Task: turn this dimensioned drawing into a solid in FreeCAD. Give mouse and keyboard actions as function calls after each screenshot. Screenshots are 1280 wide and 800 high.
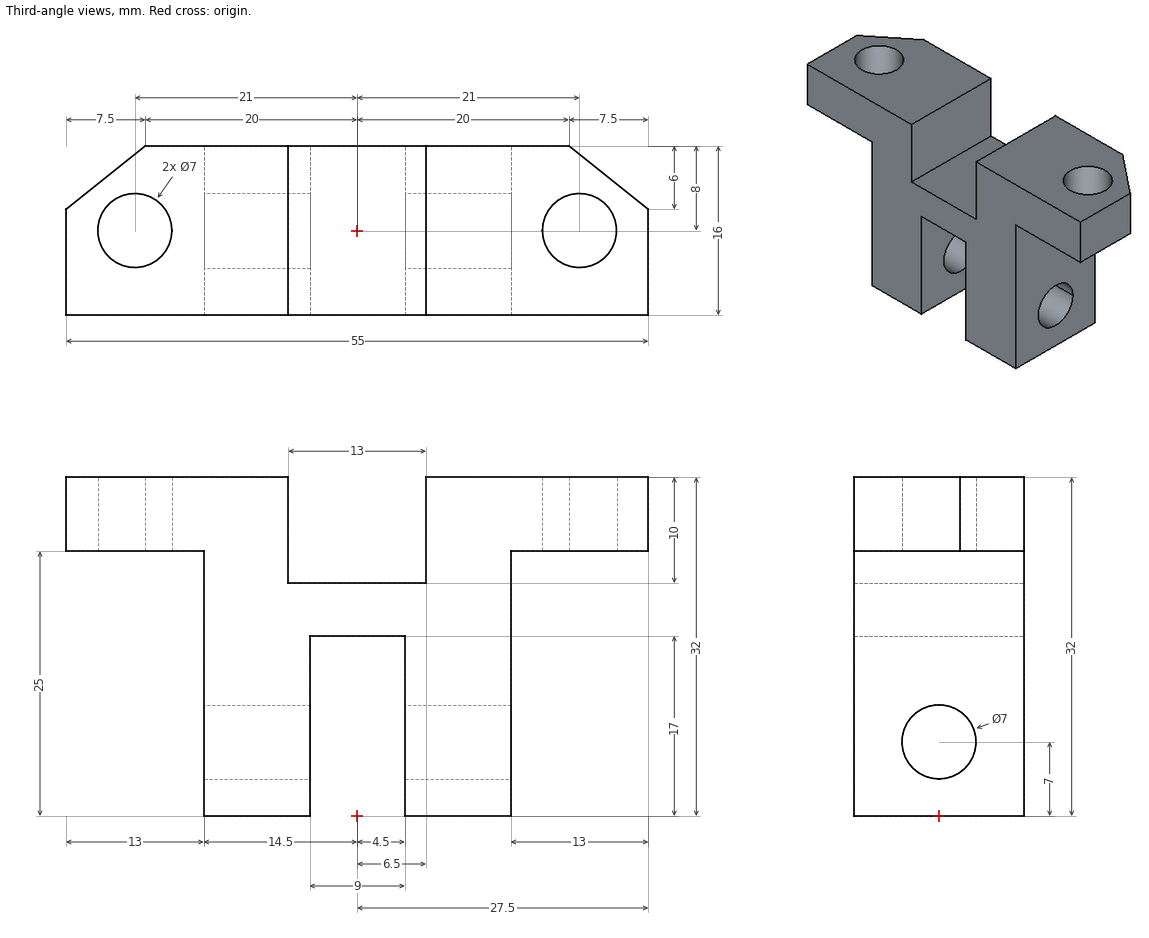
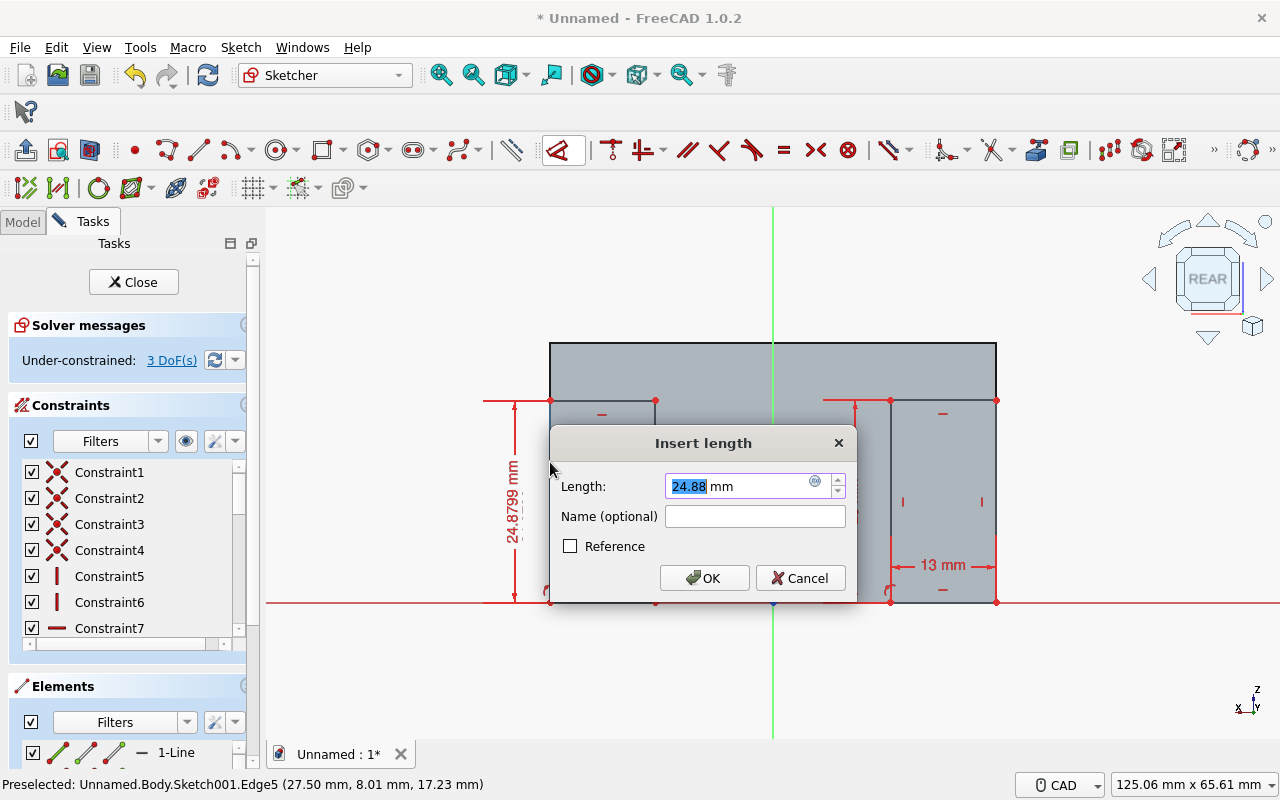
text(25)
key(Return)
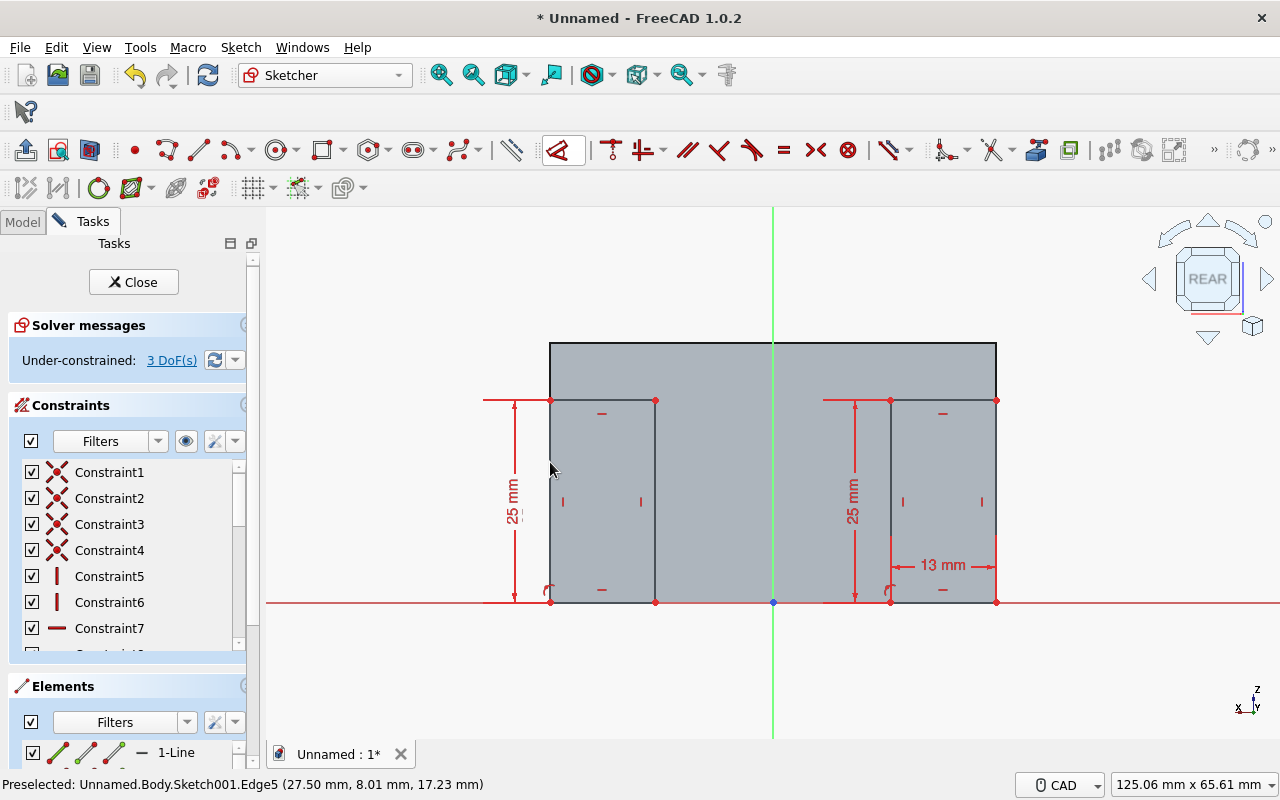
click(581, 603)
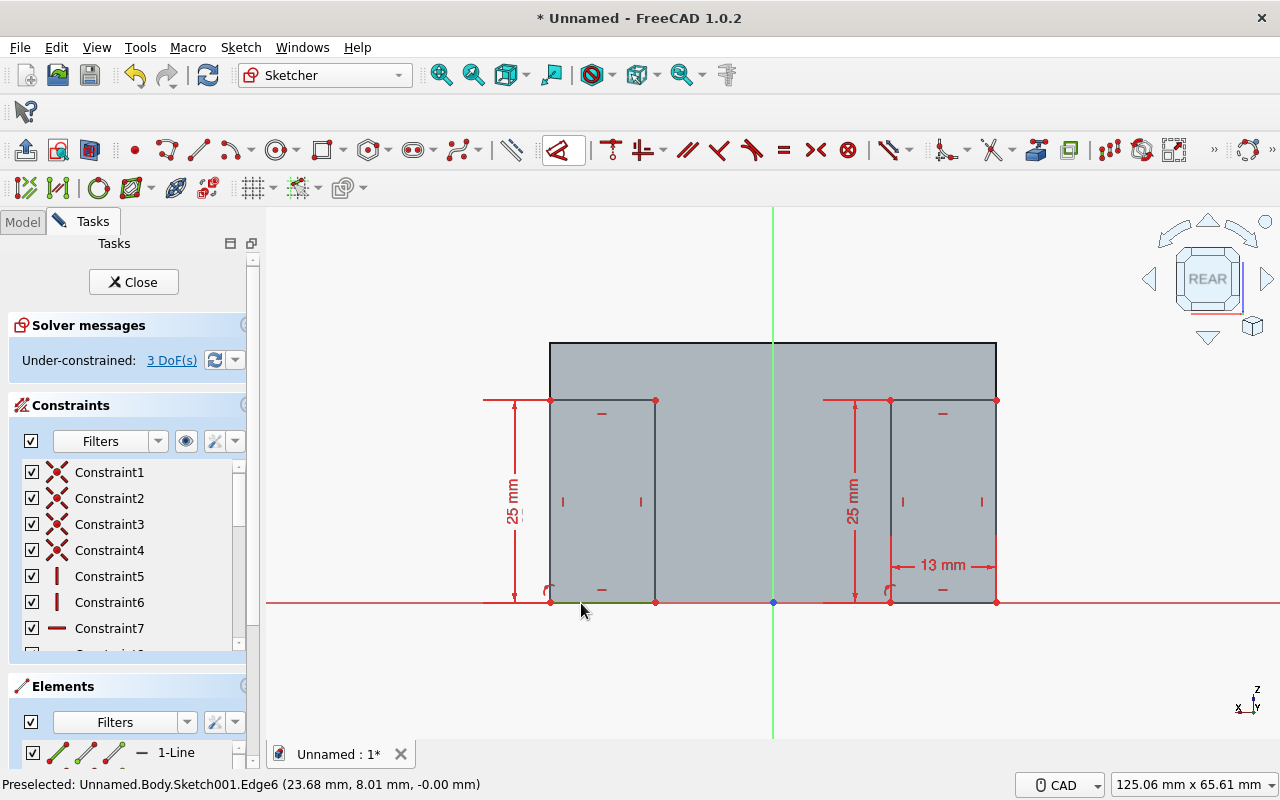
click(580, 150)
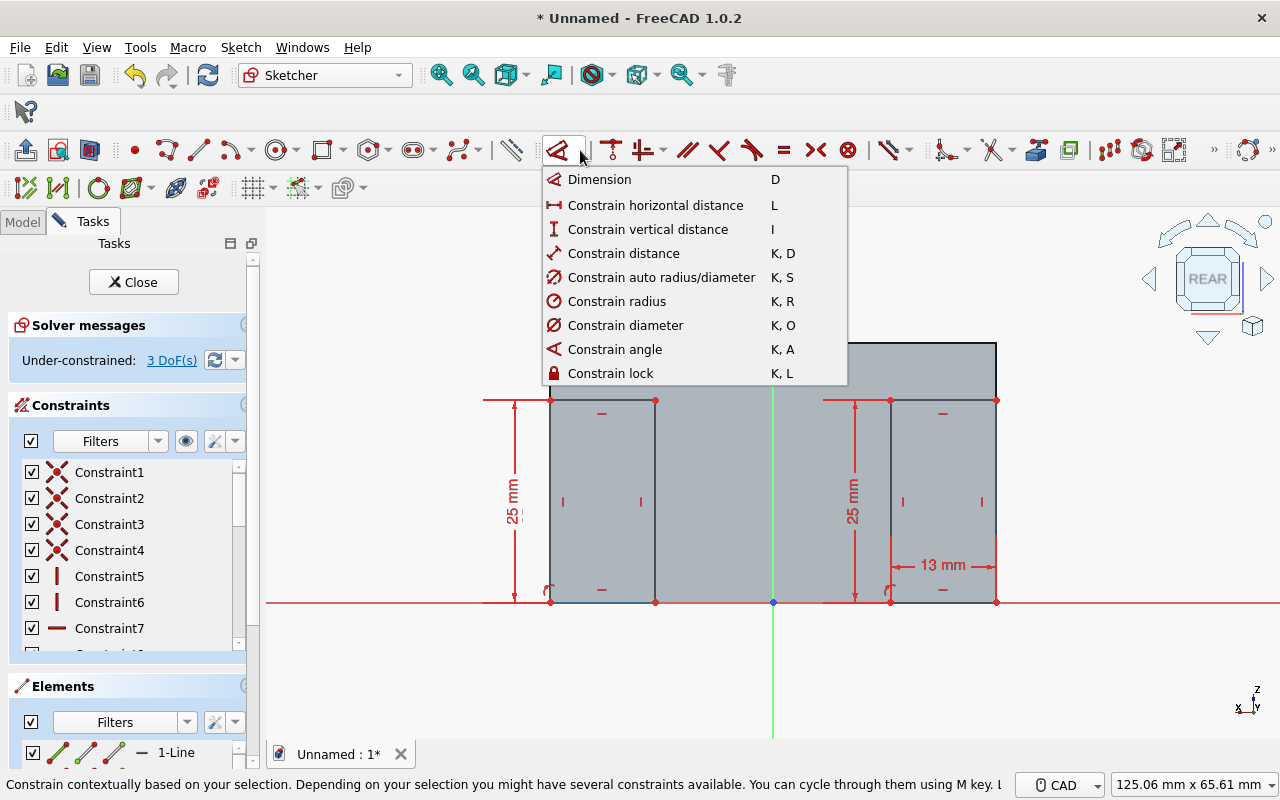
click(695, 205)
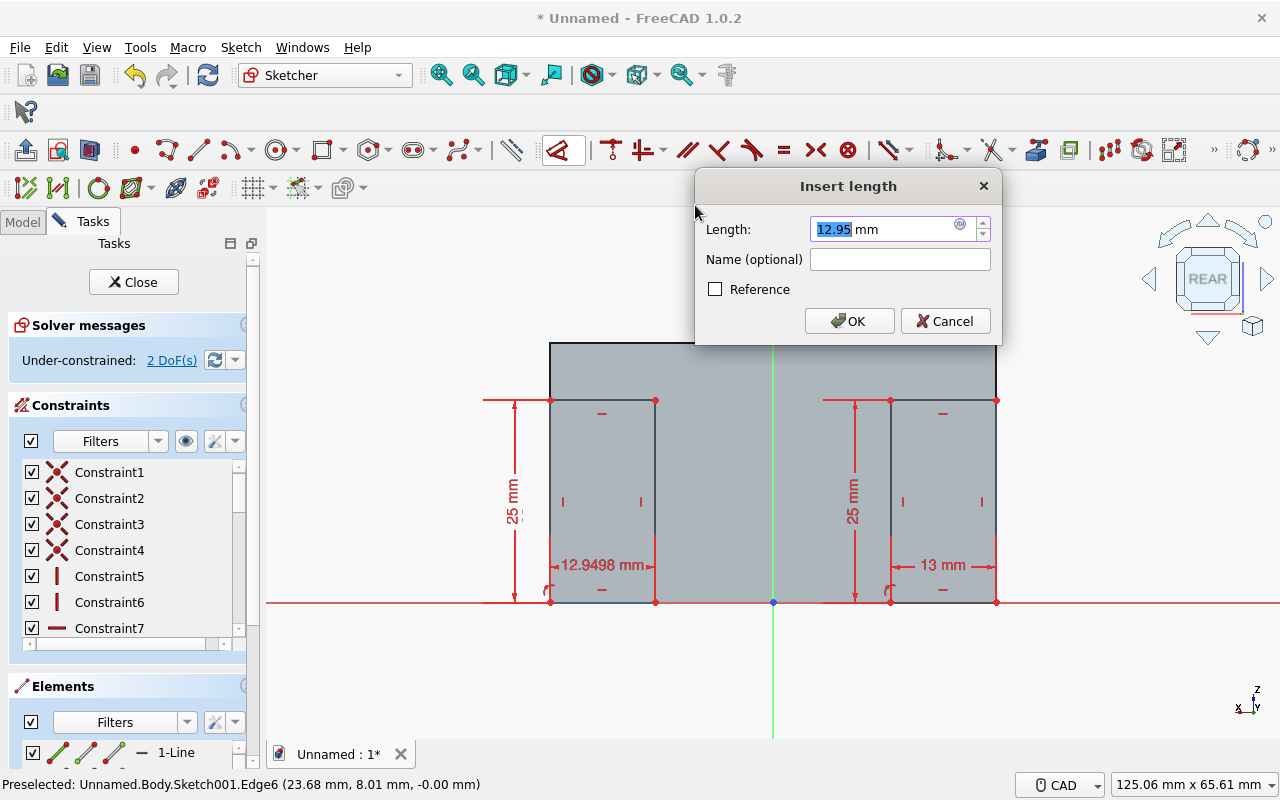
text(13)
key(Return)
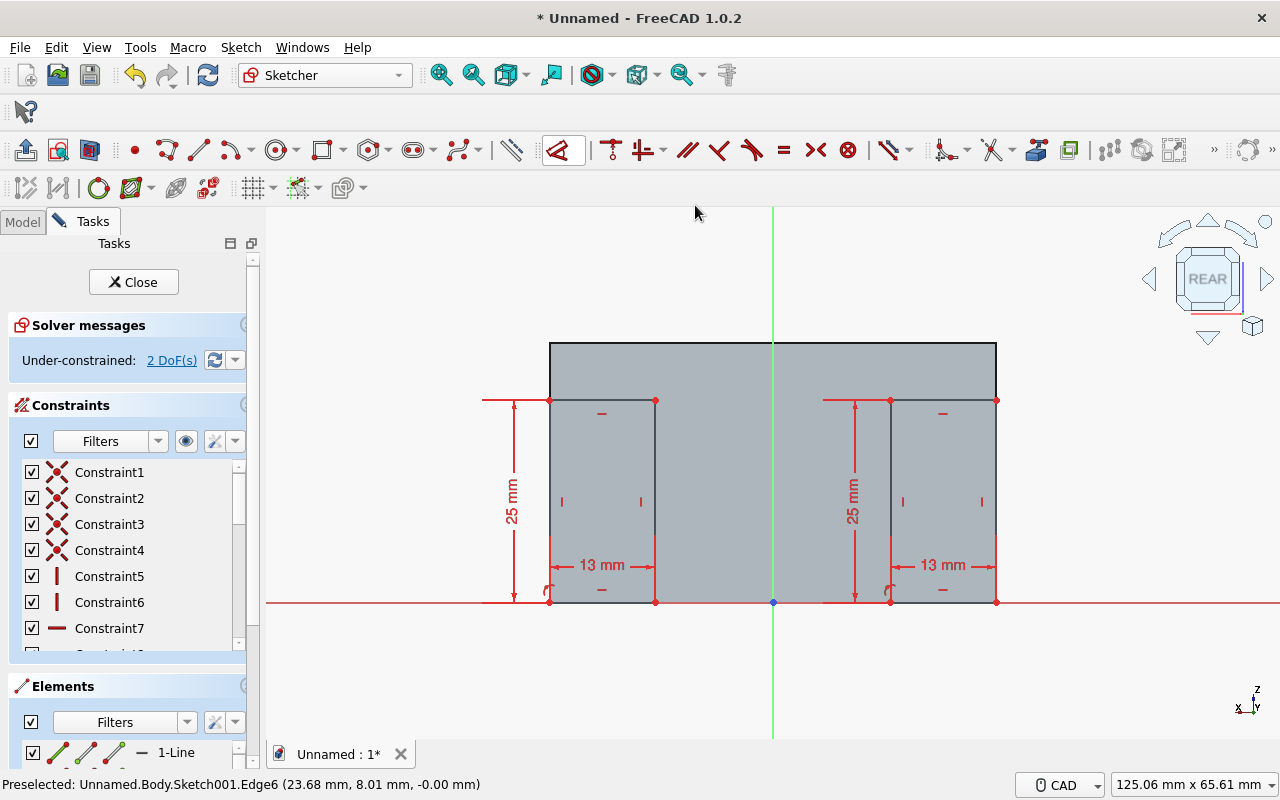
click(891, 400)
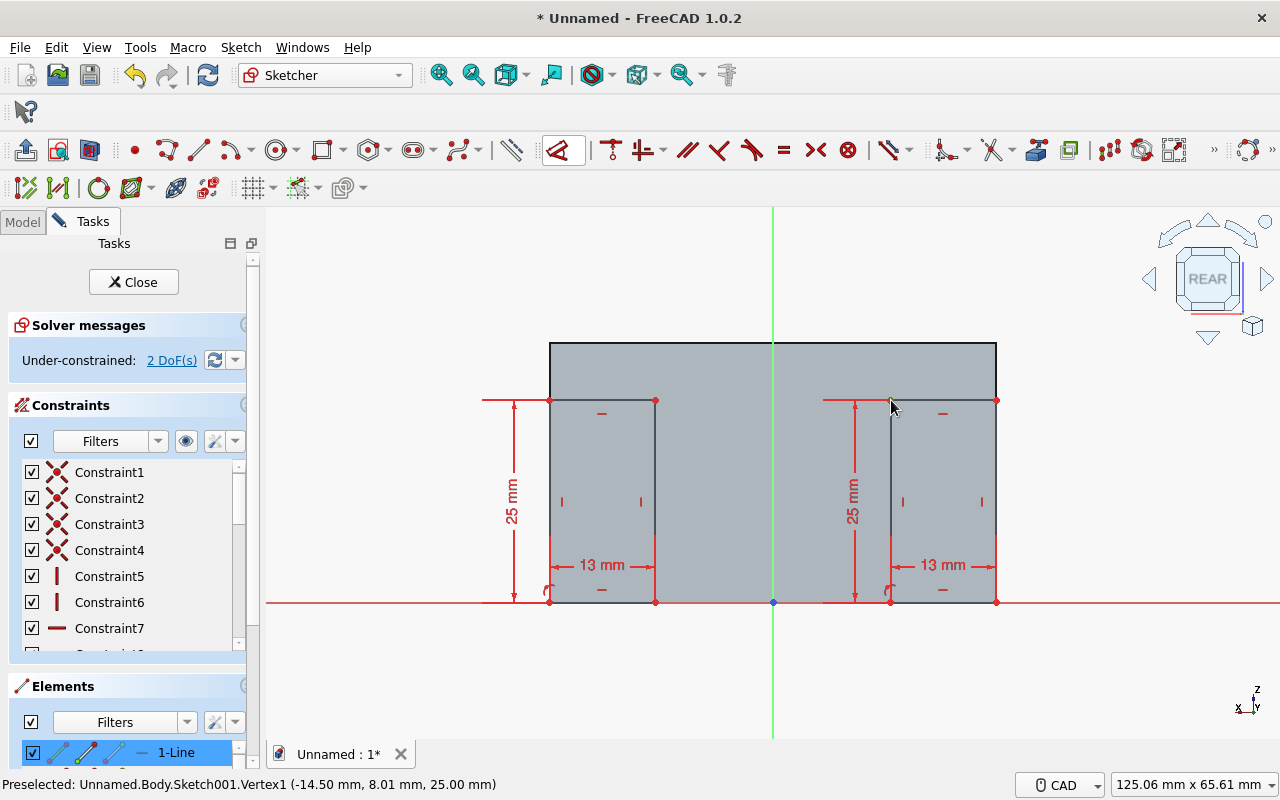
key(l)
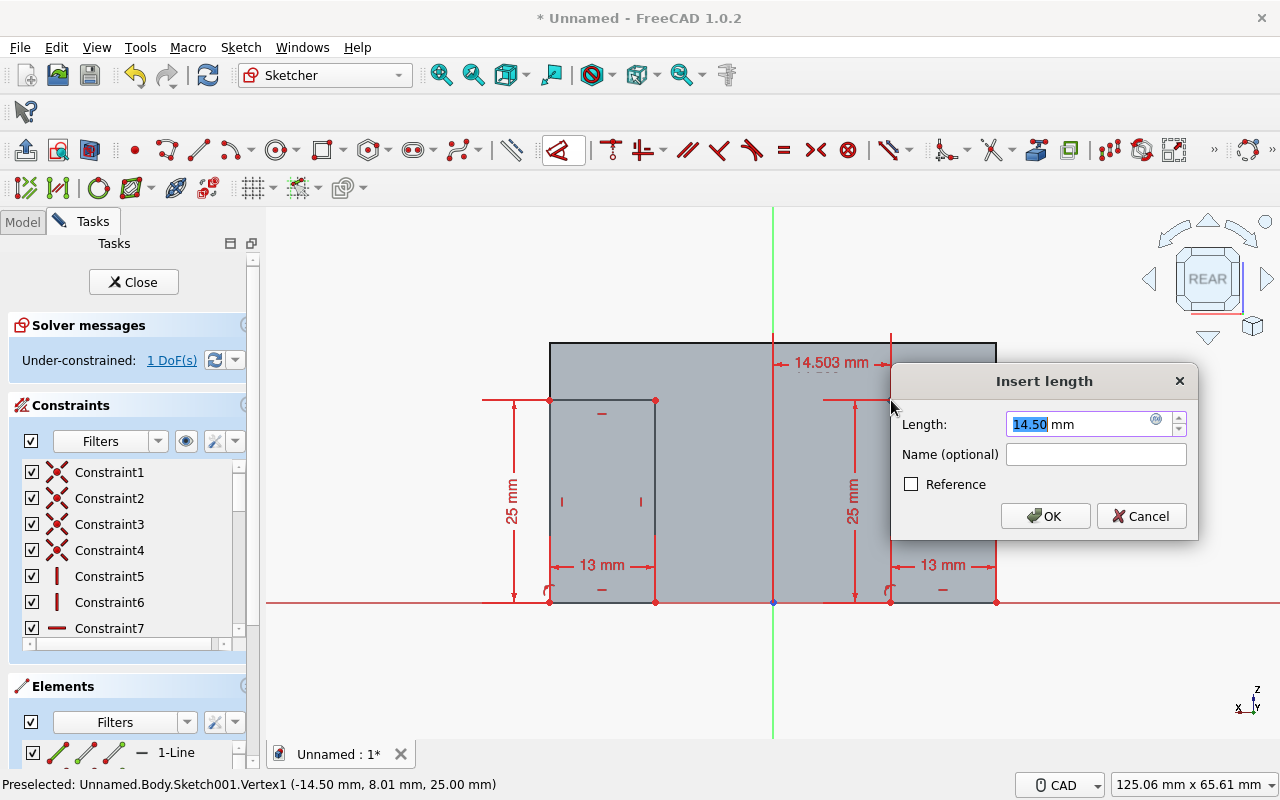
text(14.5)
key(Return)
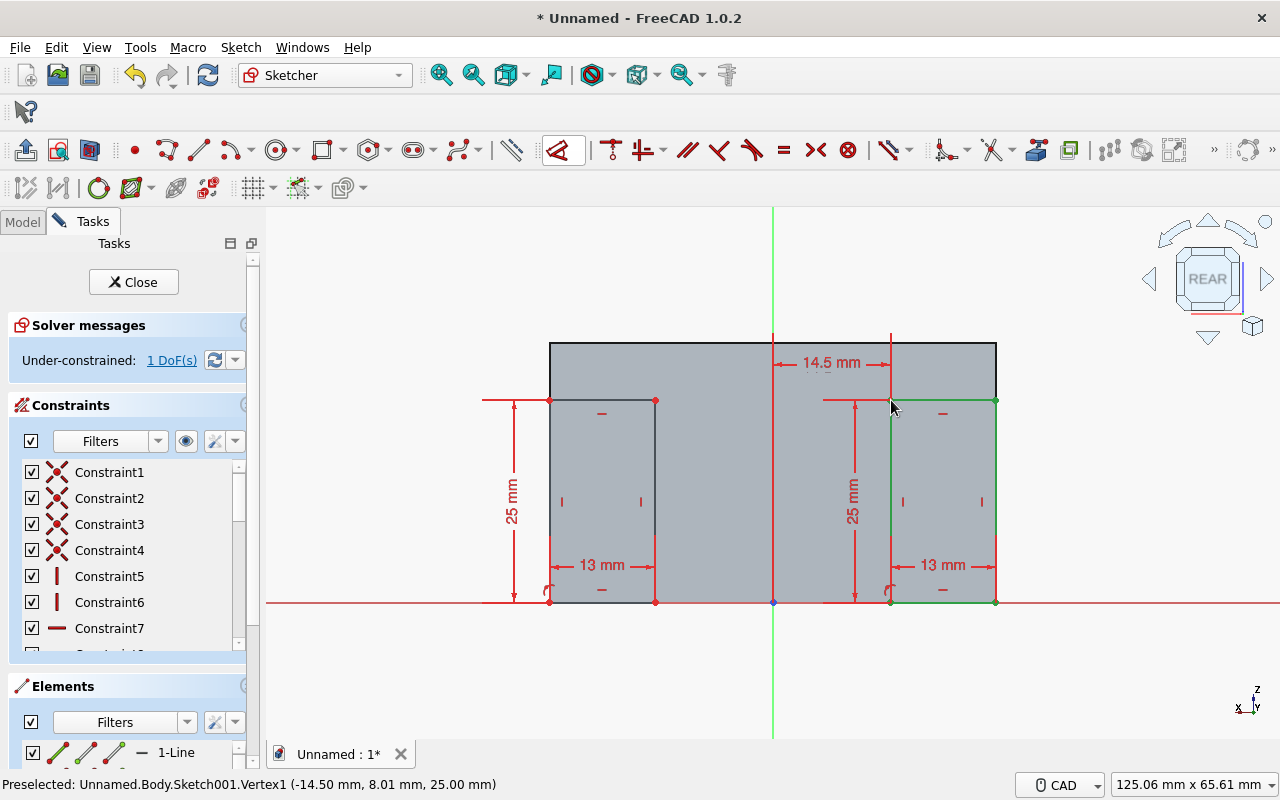
click(550, 400)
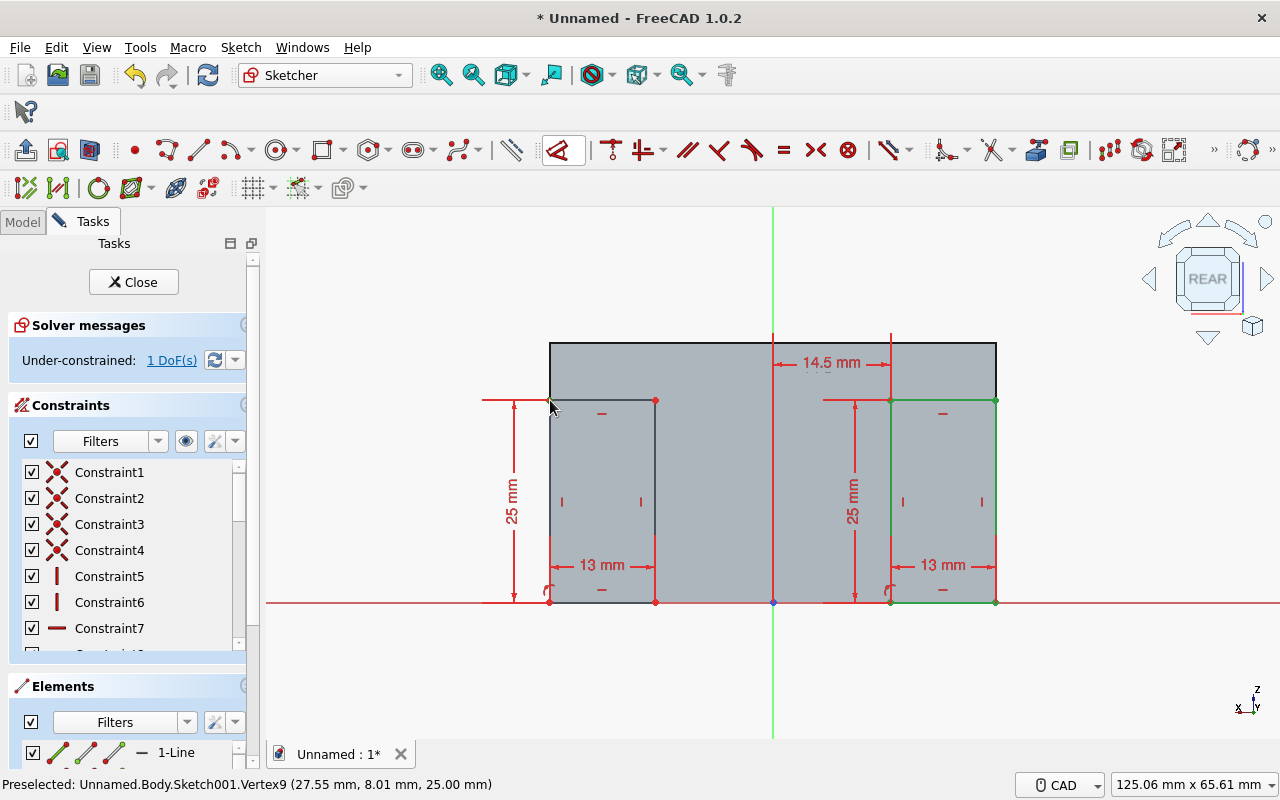
click(580, 150)